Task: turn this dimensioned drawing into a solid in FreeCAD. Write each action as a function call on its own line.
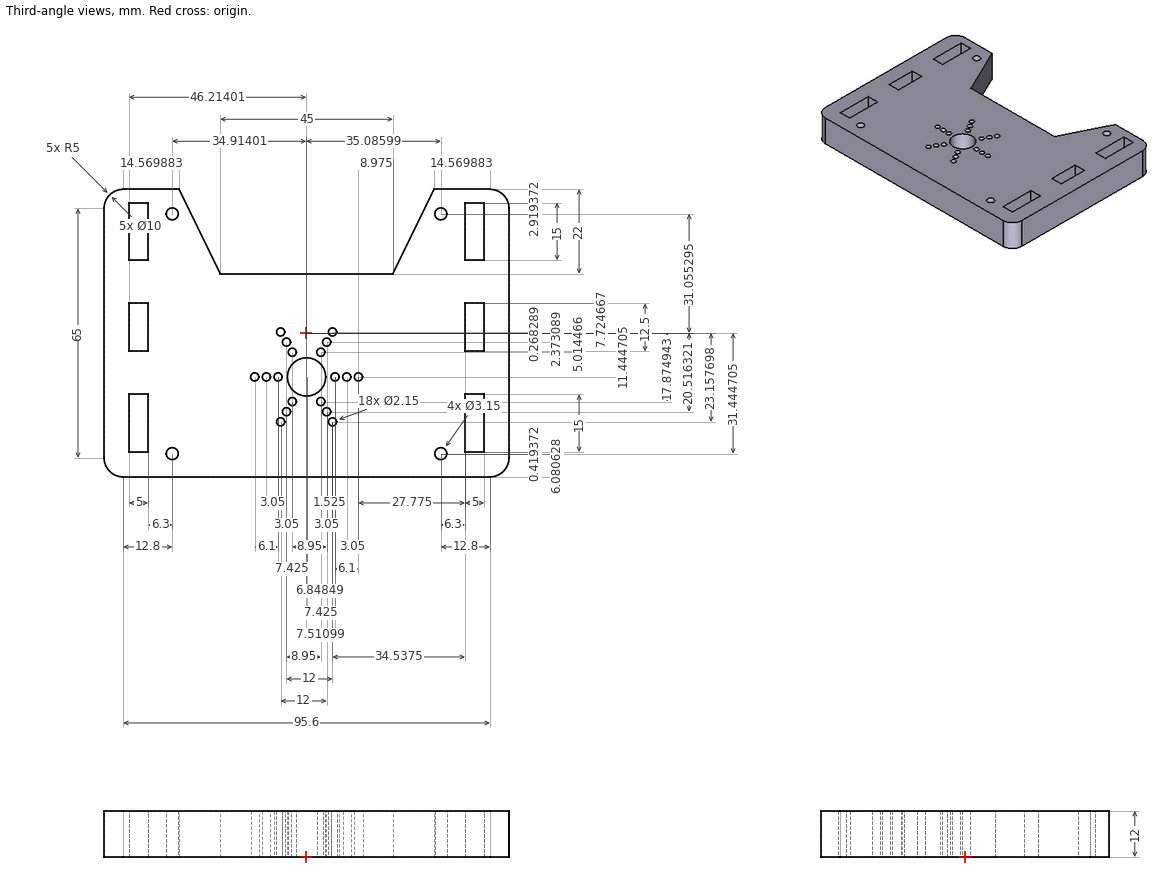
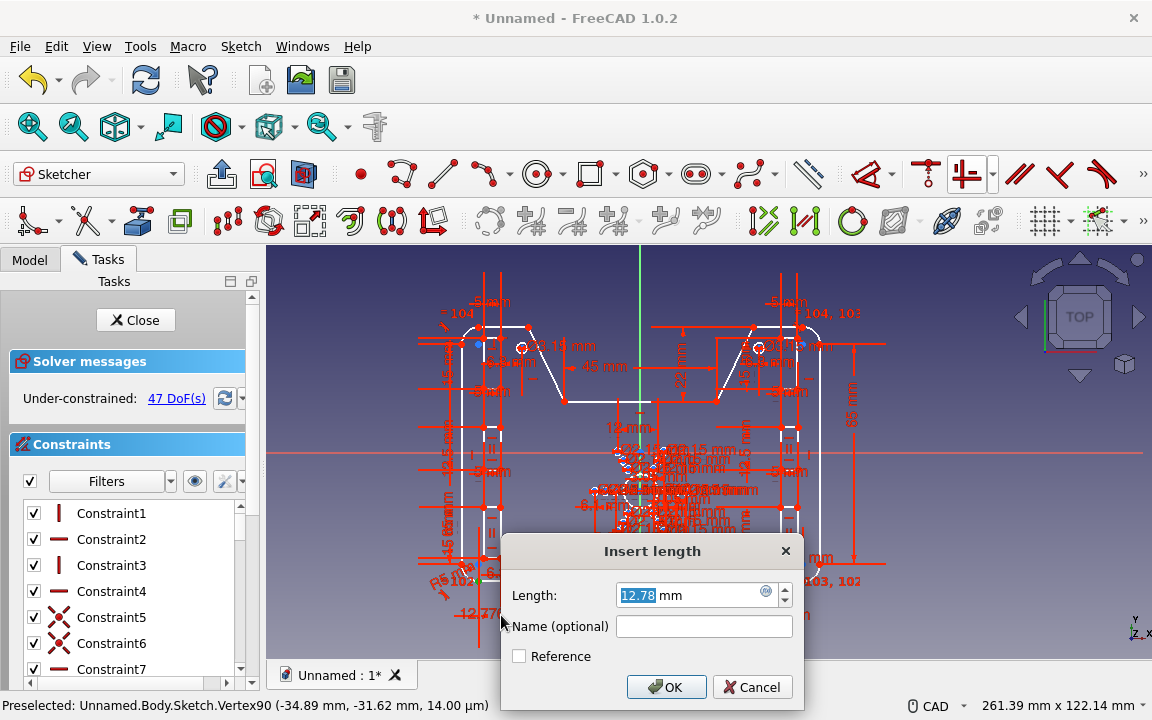
text(12.8)
key(Return)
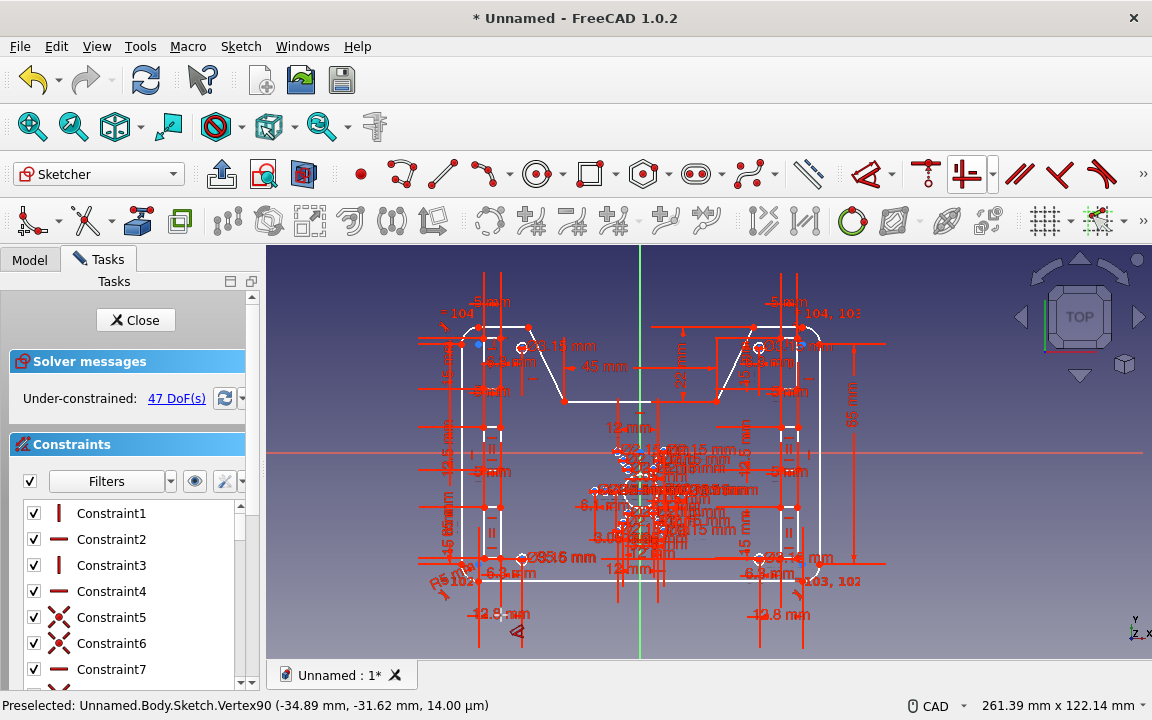
scroll(616, 492, up, 7)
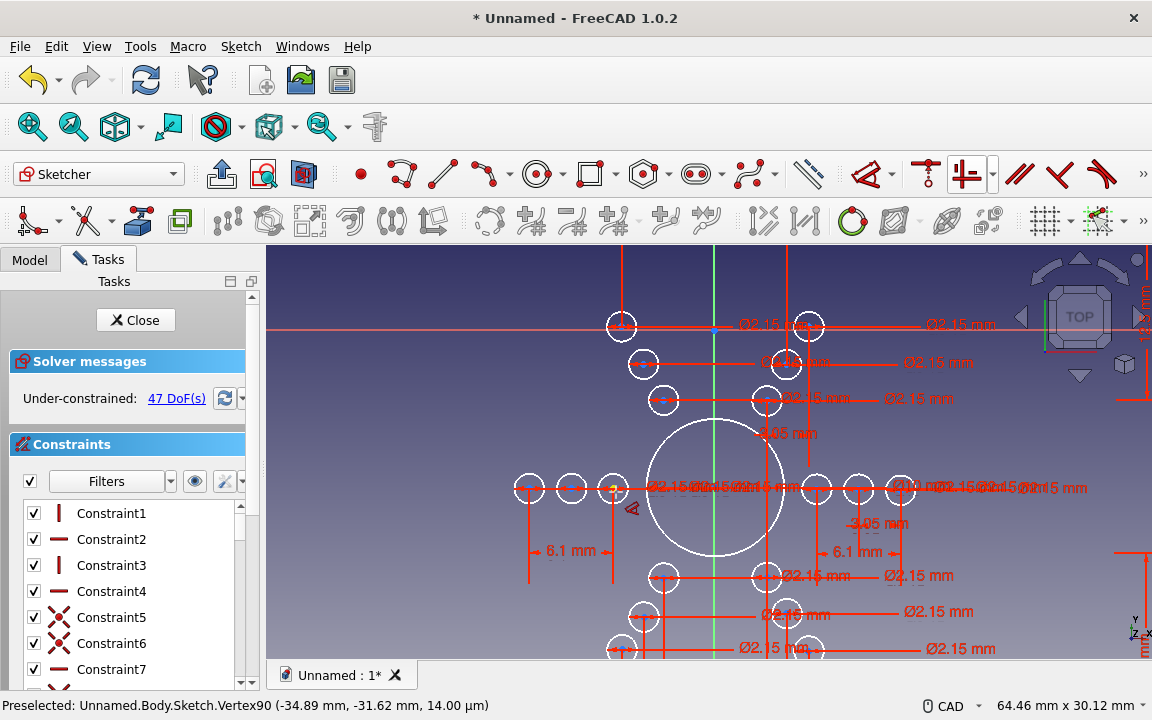
click(613, 489)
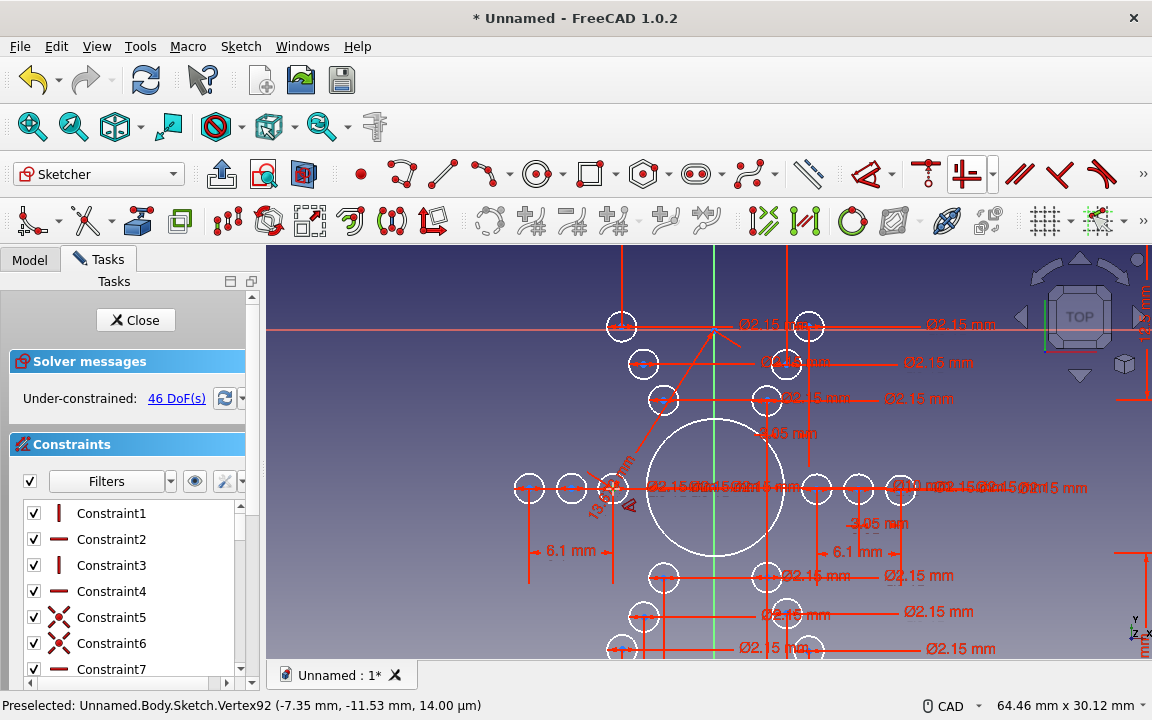
click(572, 489)
click(592, 523)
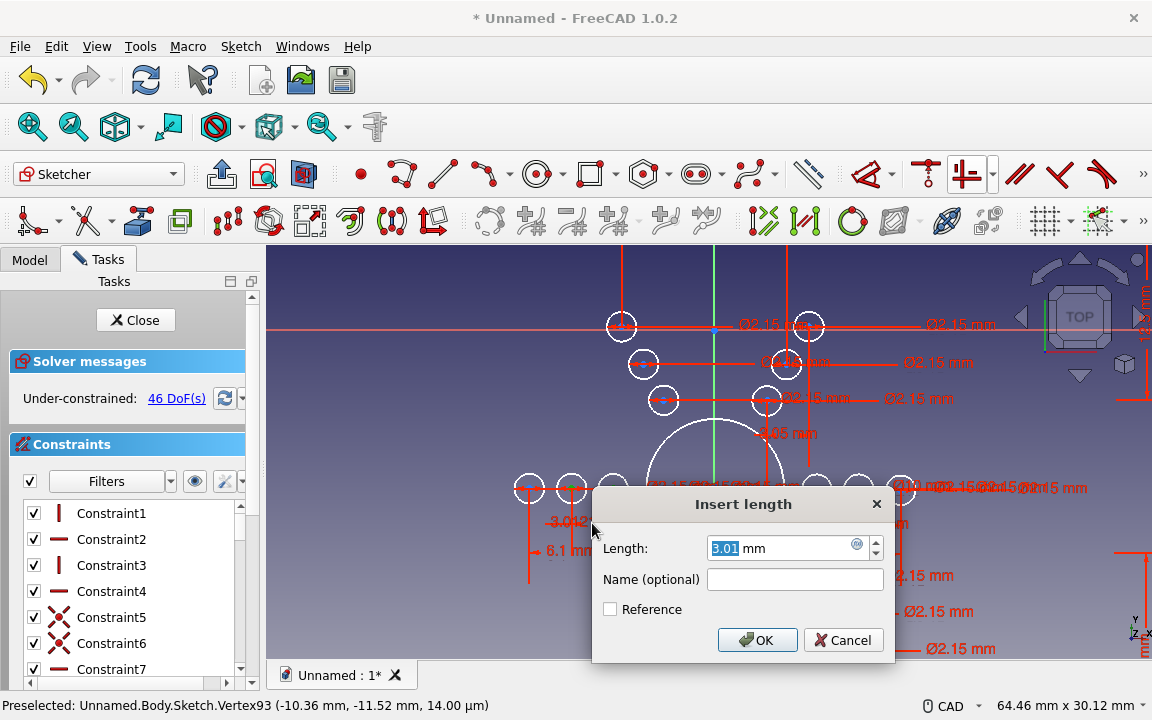
text(3.05)
key(Return)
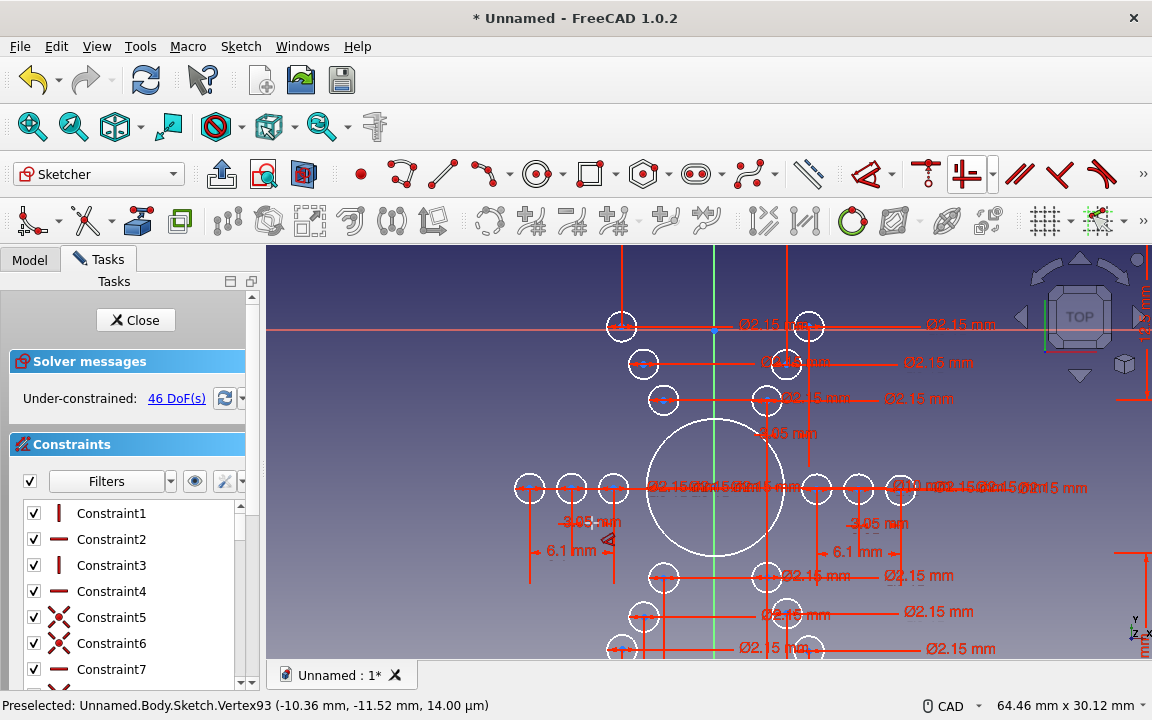
scroll(616, 492, down, 7)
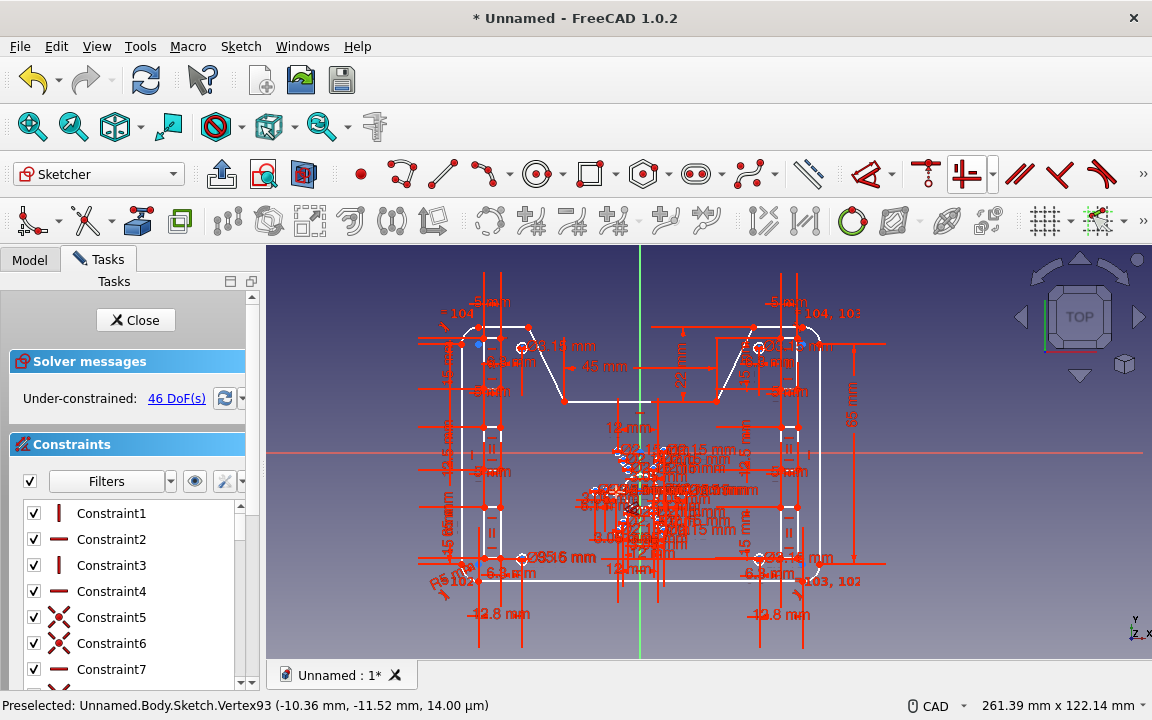
scroll(658, 461, up, 2)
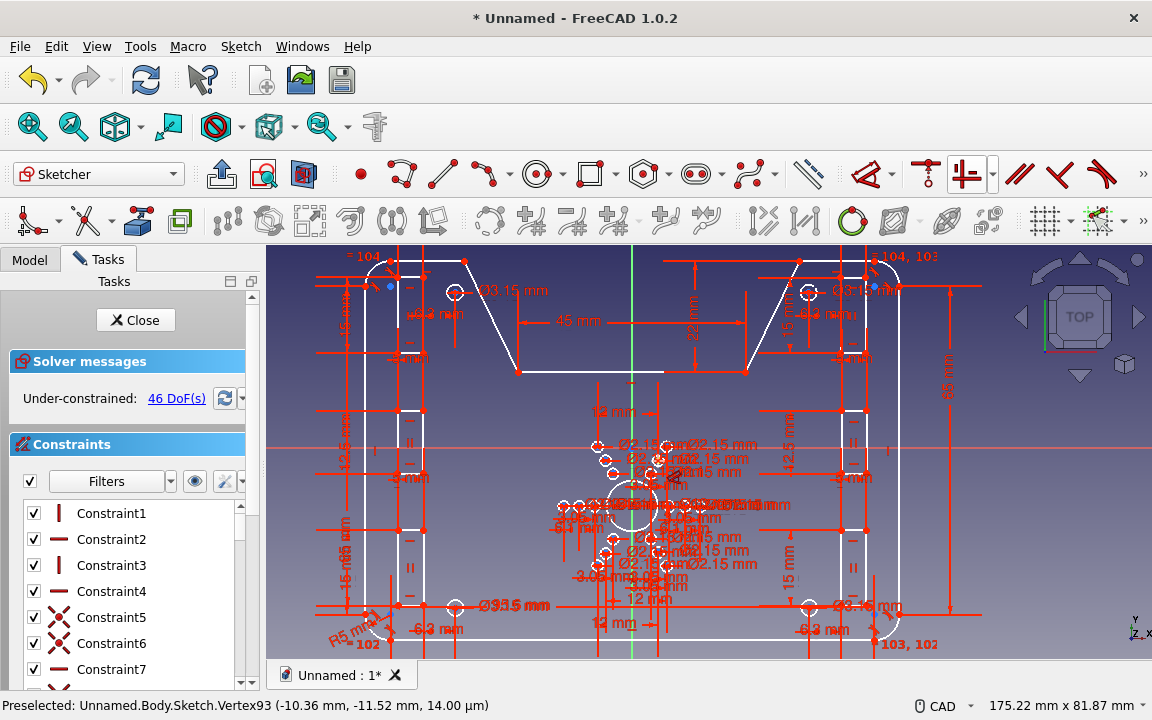
click(658, 461)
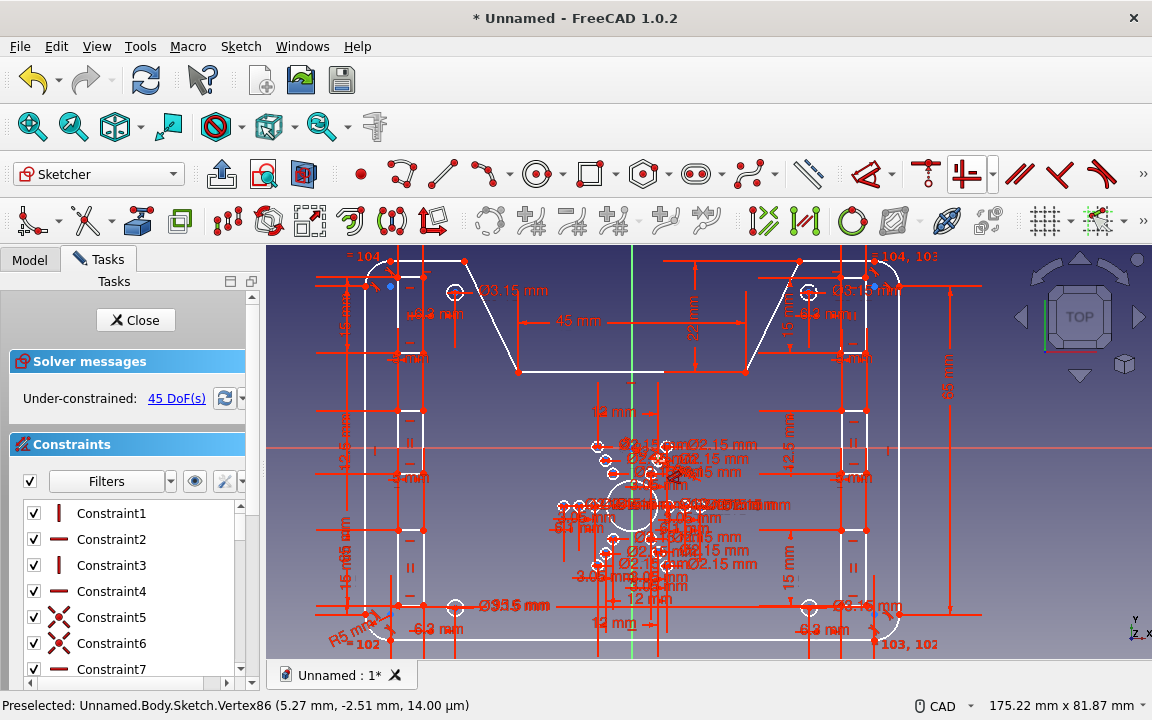
click(613, 474)
click(646, 355)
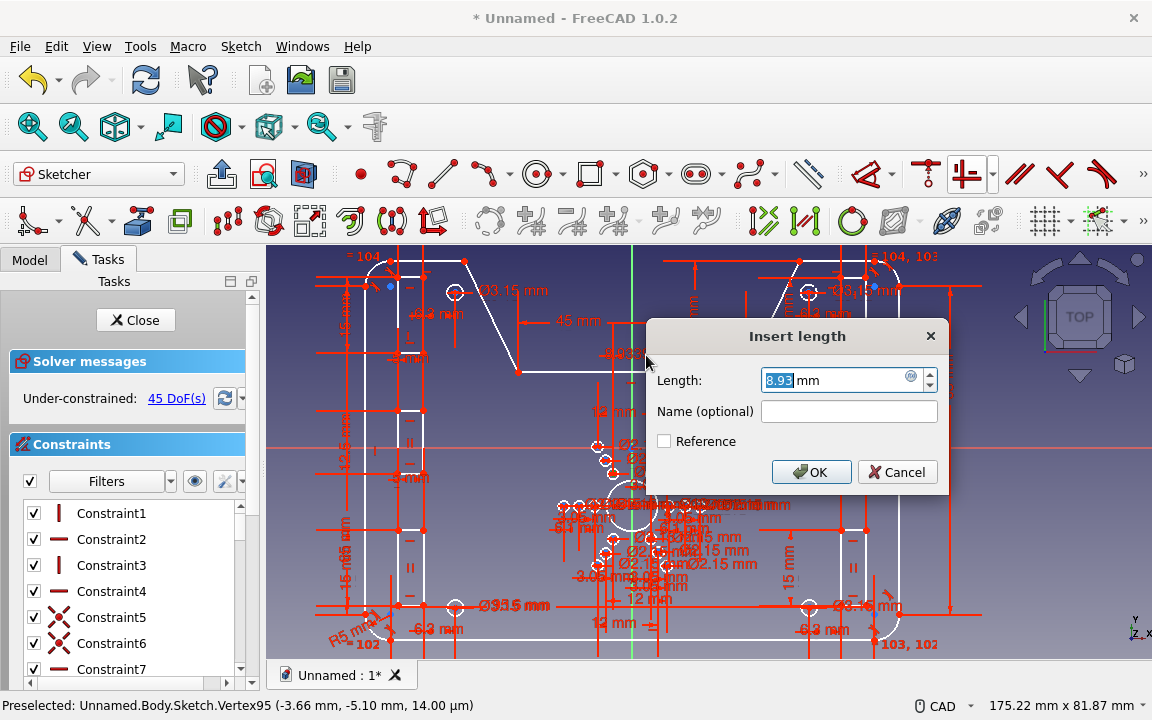
text(8.95)
key(Return)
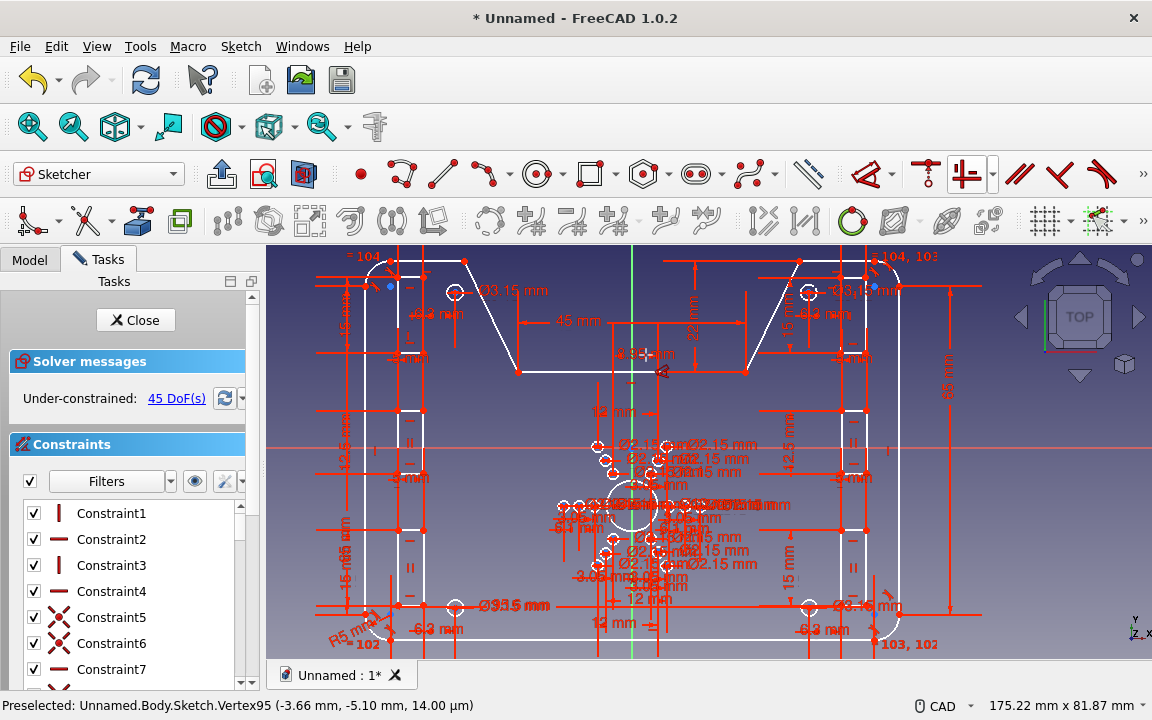
click(651, 474)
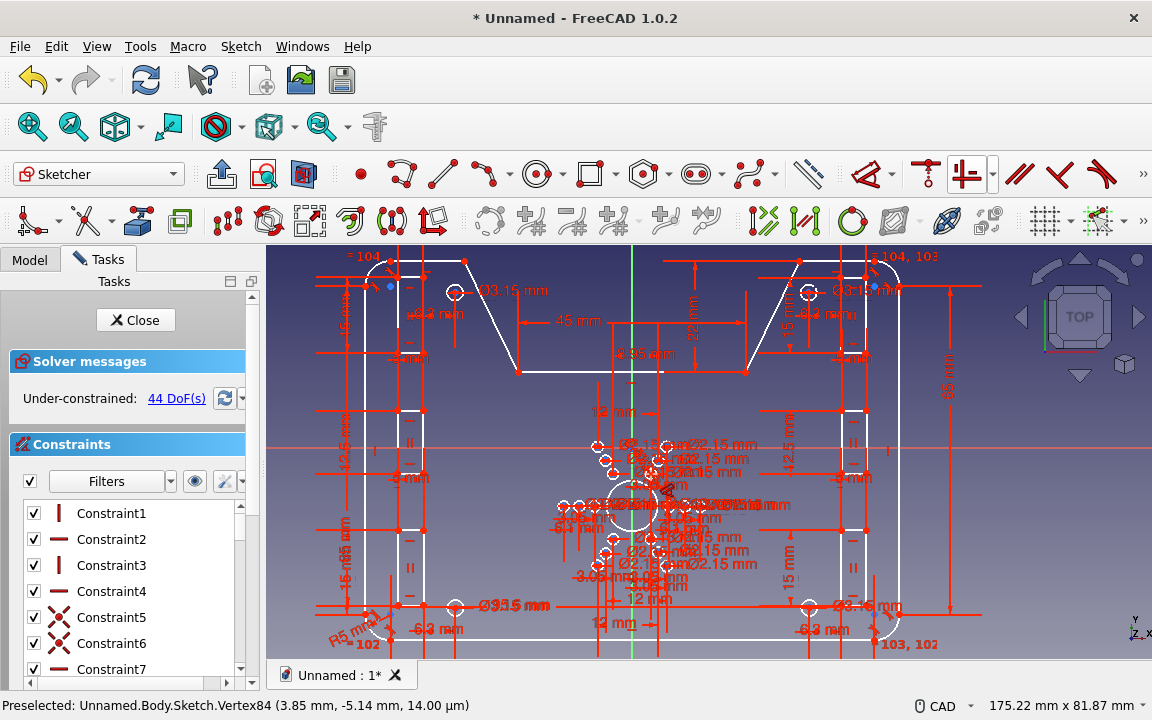
click(606, 461)
click(618, 281)